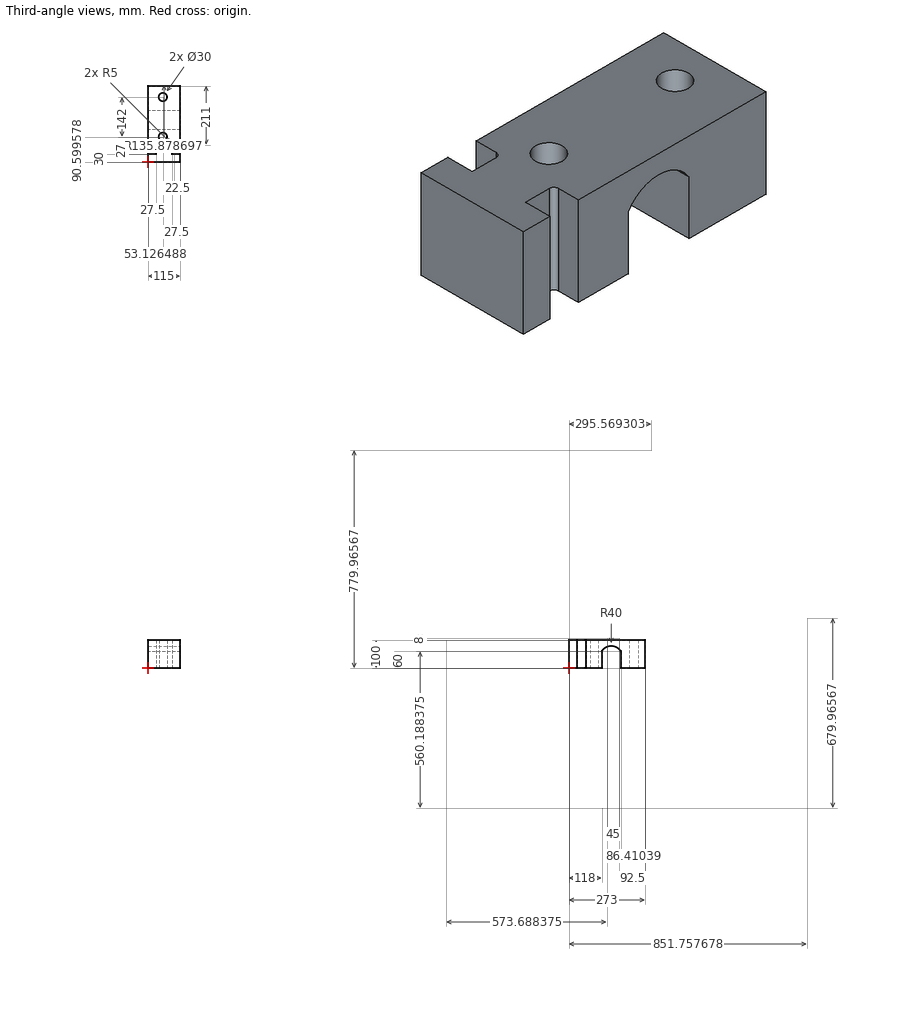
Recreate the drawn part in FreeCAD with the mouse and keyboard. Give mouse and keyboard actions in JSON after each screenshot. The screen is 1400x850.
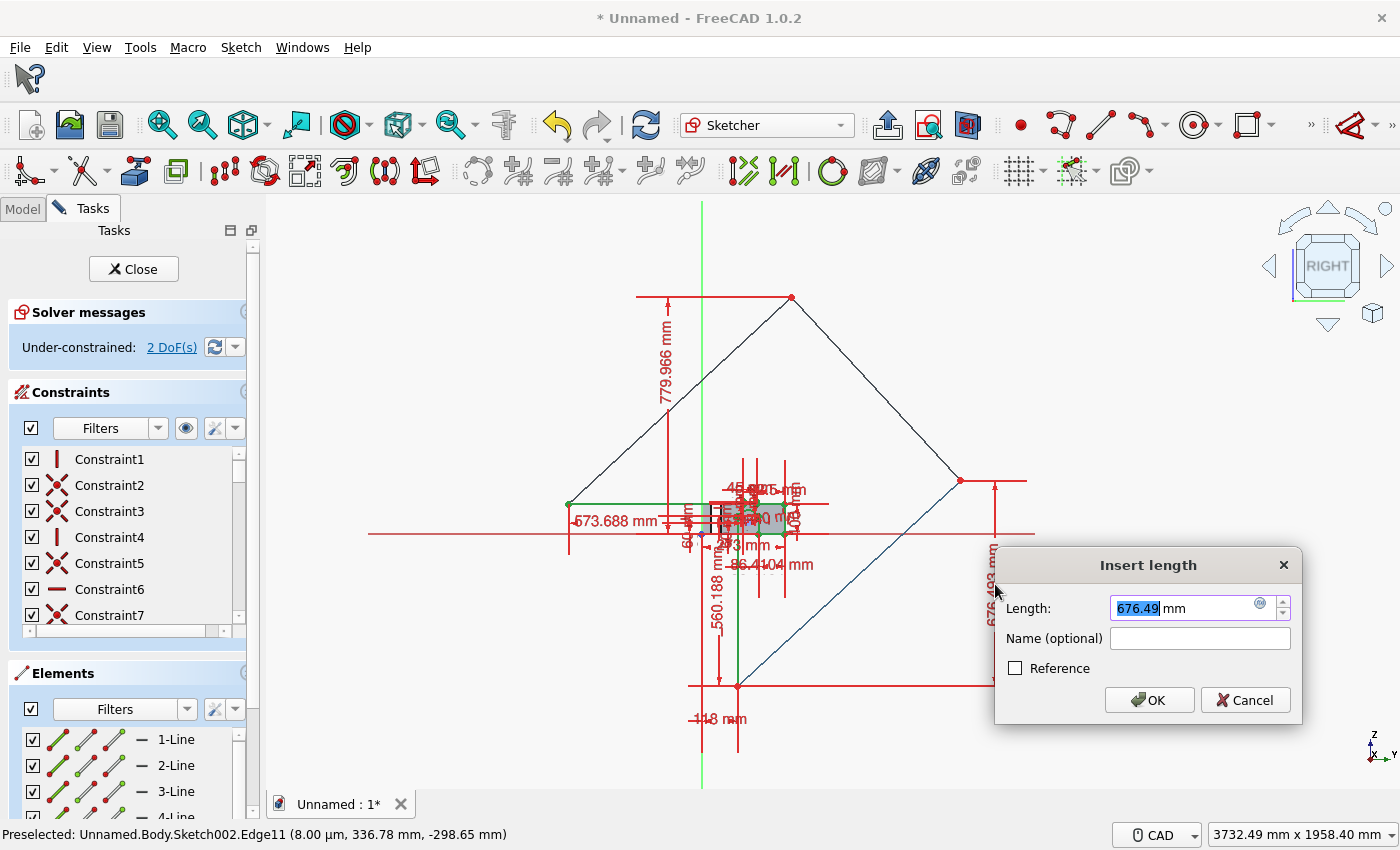
{"action": "type", "text": "679.96567"}
{"action": "key", "text": "Return"}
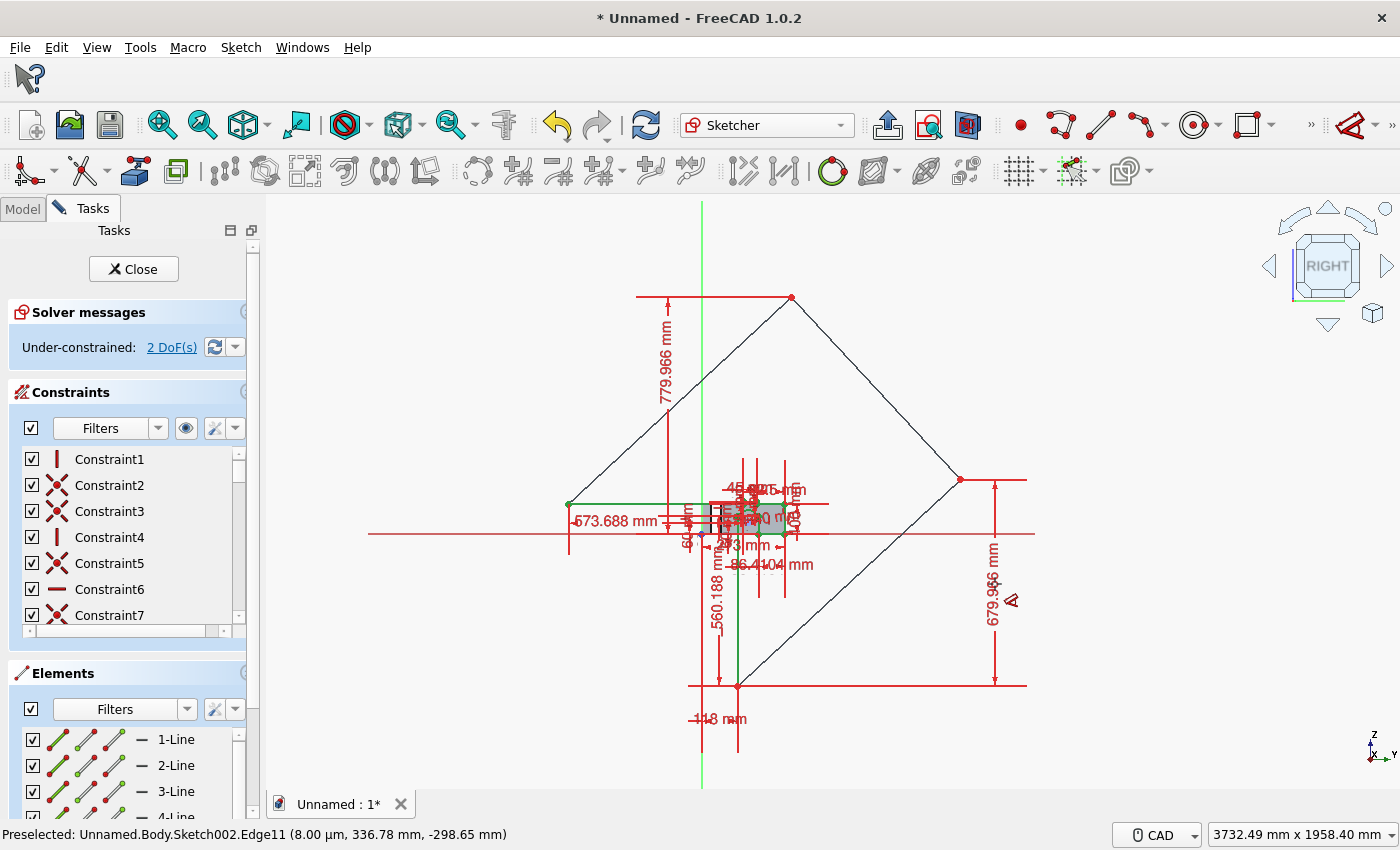
{"action": "left_click", "coordinate": [791, 297]}
{"action": "left_click", "coordinate": [747, 263]}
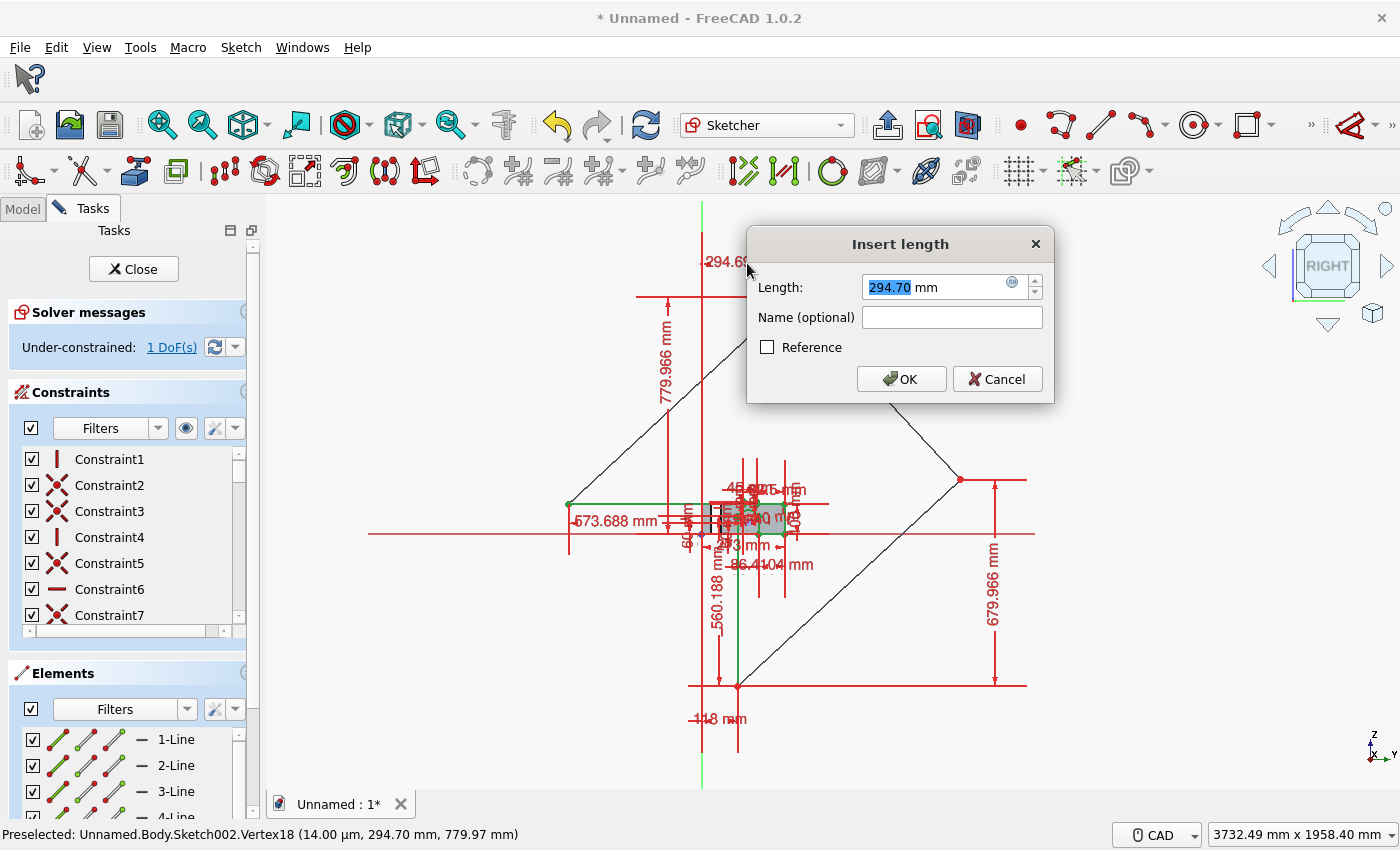
{"action": "type", "text": "295.569303"}
{"action": "key", "text": "Return"}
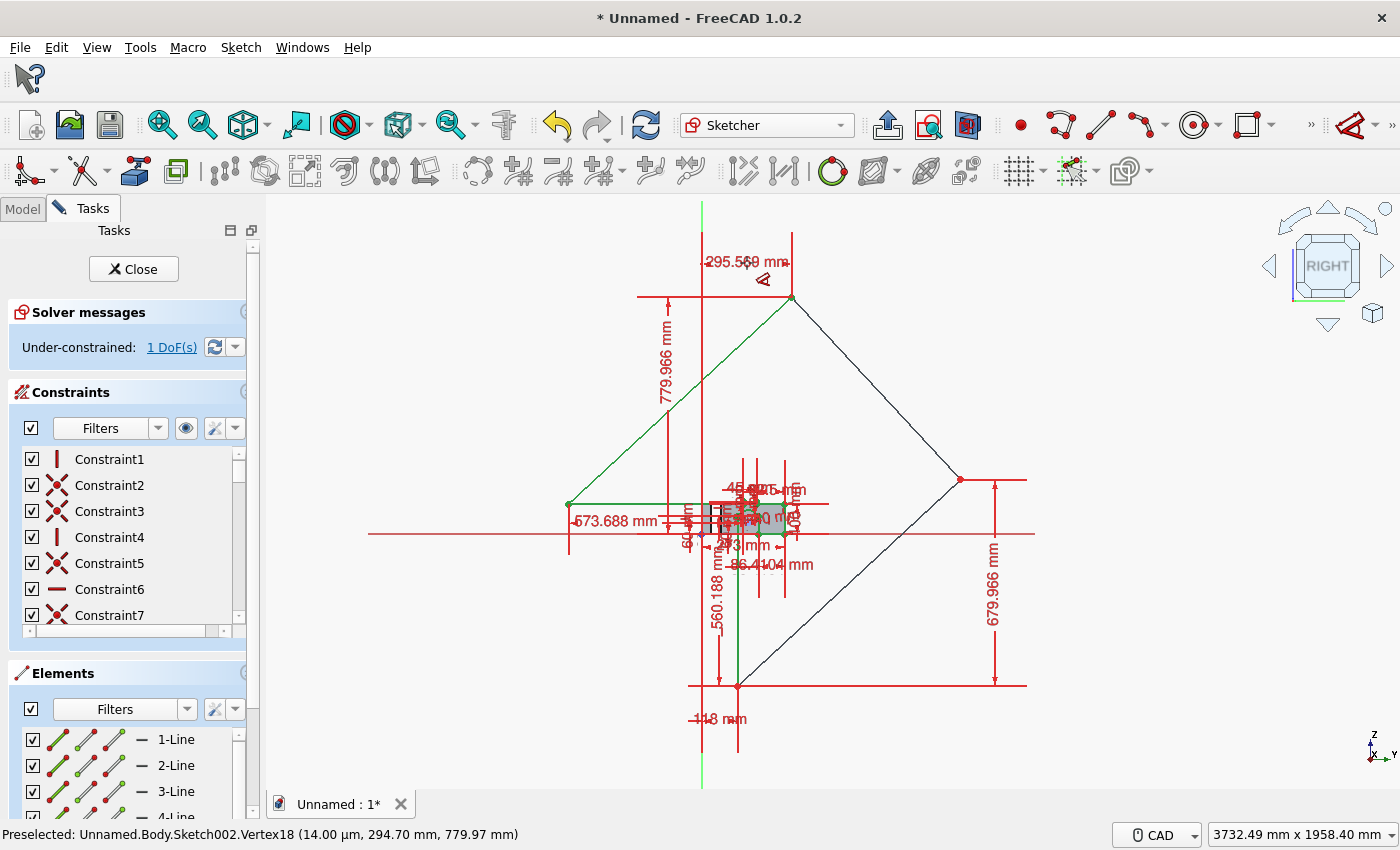
{"action": "left_click", "coordinate": [961, 480]}
{"action": "left_click", "coordinate": [891, 568]}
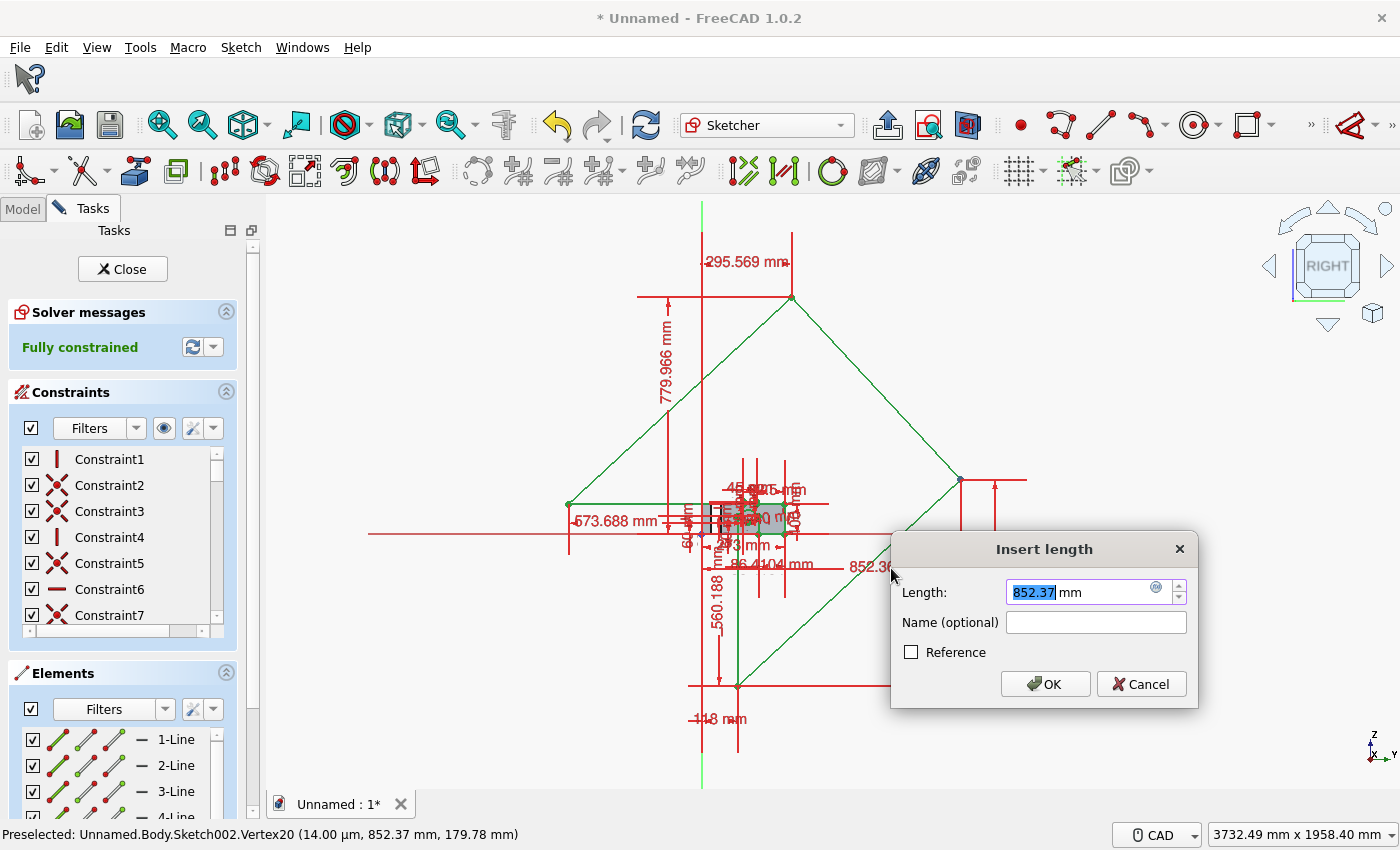
{"action": "type", "text": "851.757678"}
{"action": "key", "text": "Return"}
{"action": "key", "text": "Escape"}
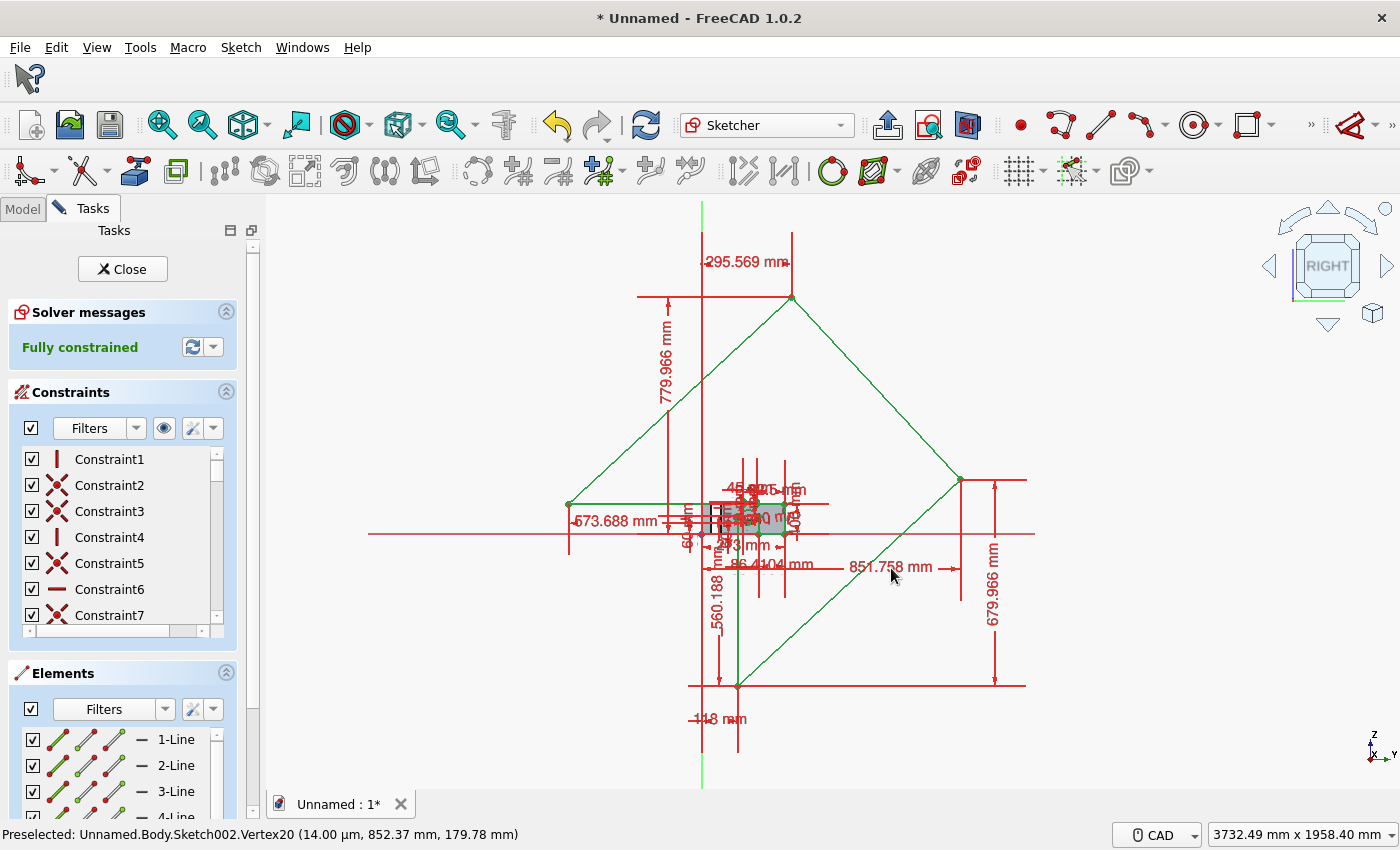
{"action": "left_click", "coordinate": [123, 269]}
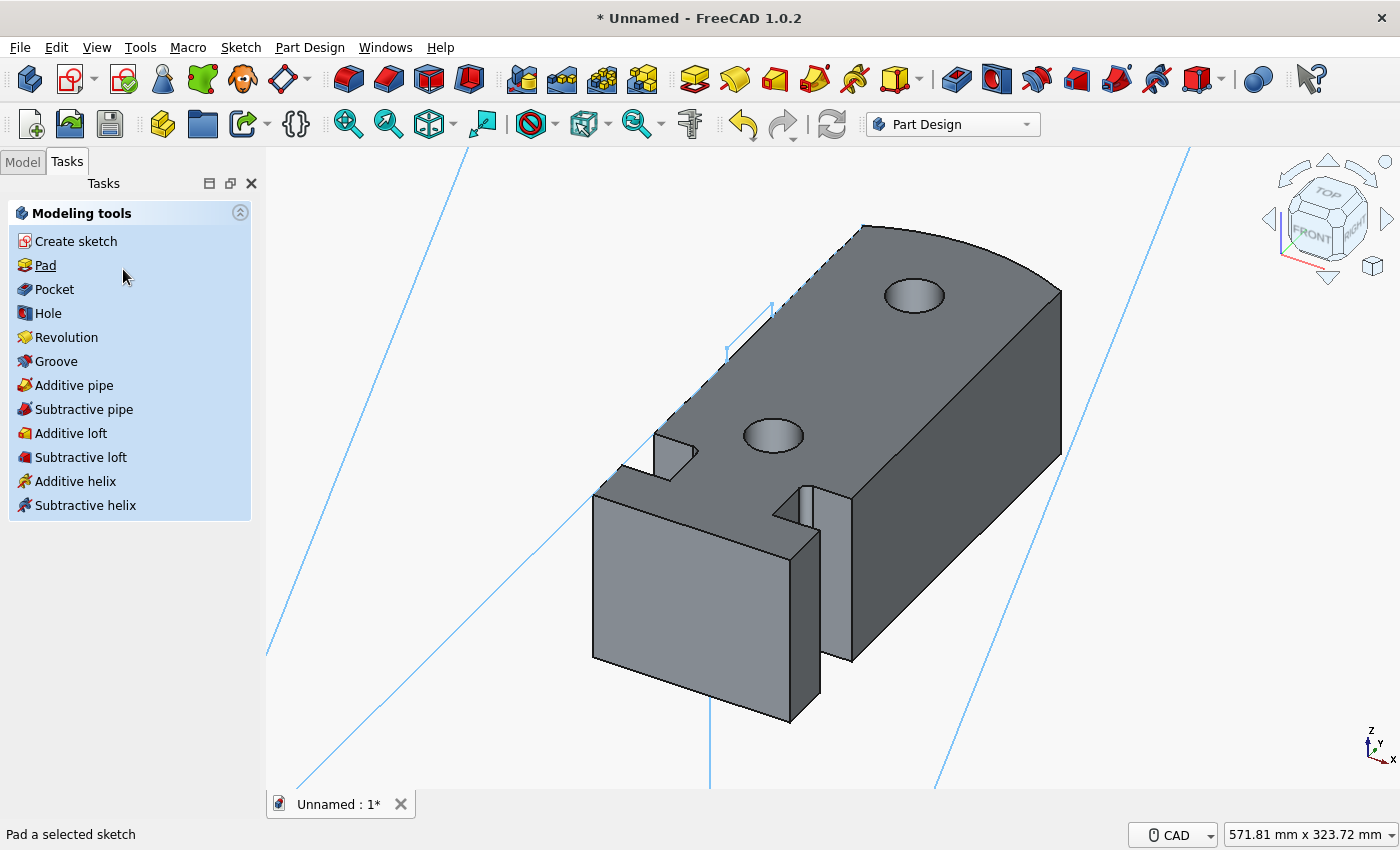
{"action": "left_click", "coordinate": [958, 80]}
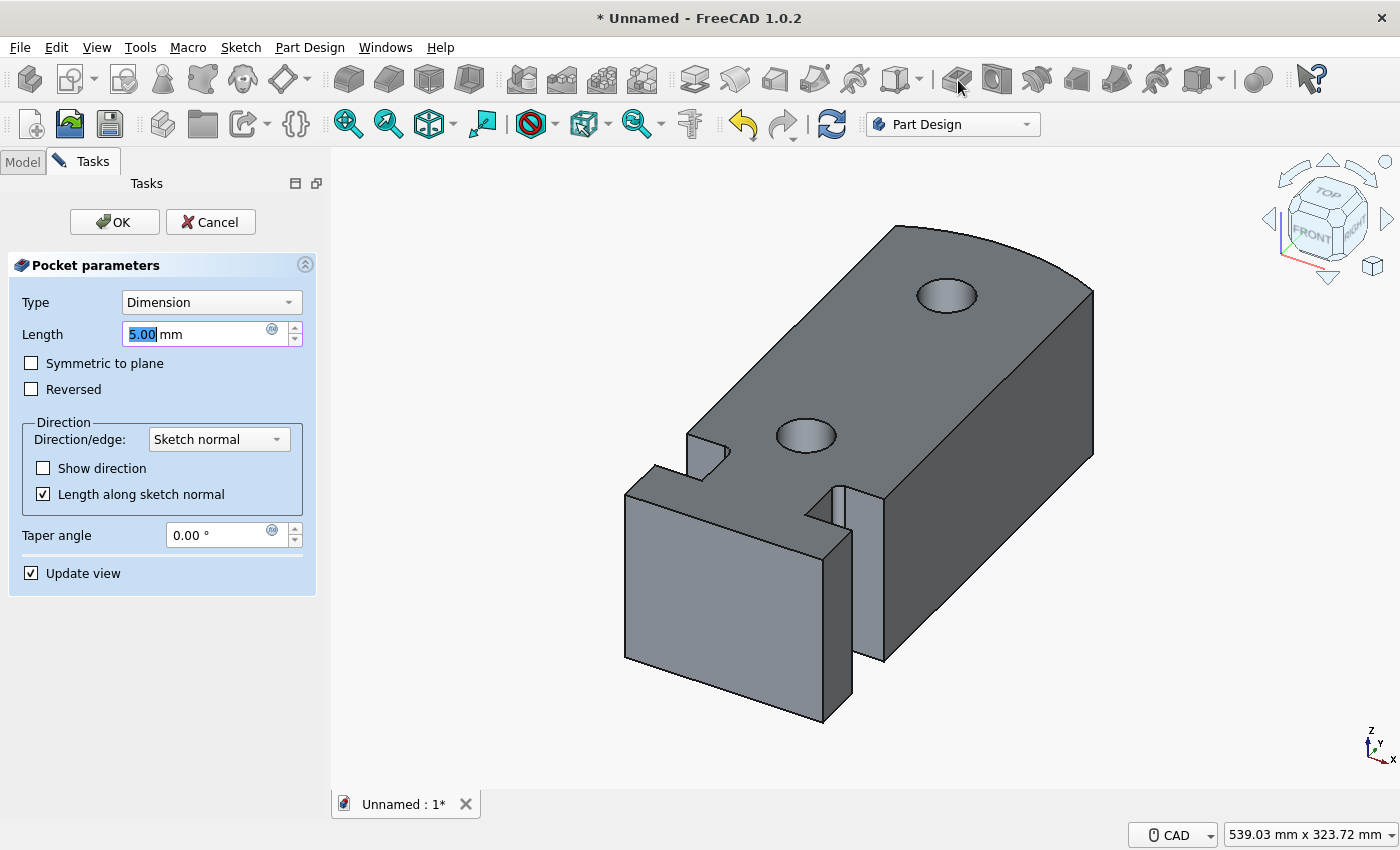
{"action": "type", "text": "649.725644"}
{"action": "key", "text": "Tab"}